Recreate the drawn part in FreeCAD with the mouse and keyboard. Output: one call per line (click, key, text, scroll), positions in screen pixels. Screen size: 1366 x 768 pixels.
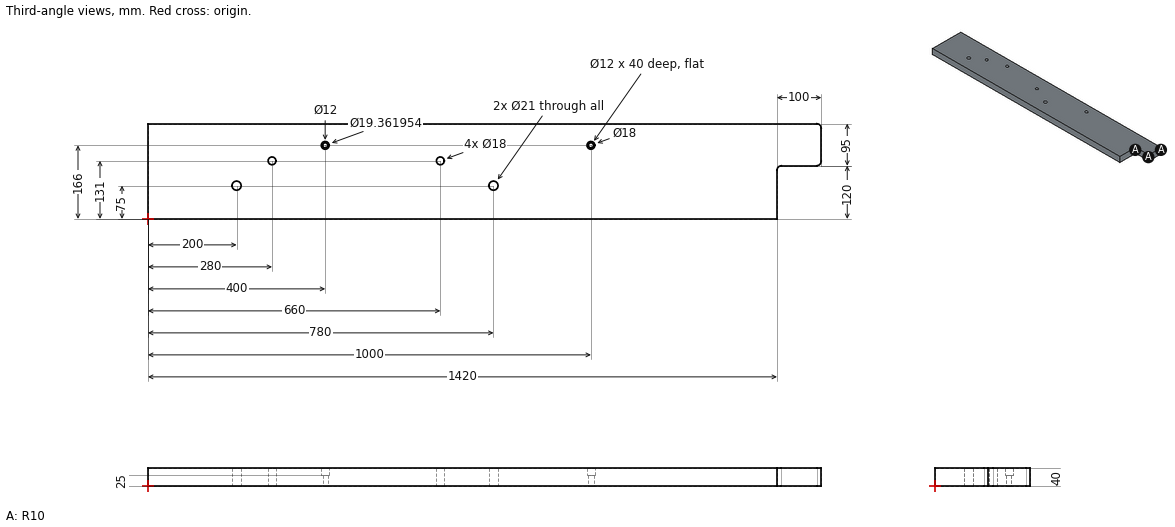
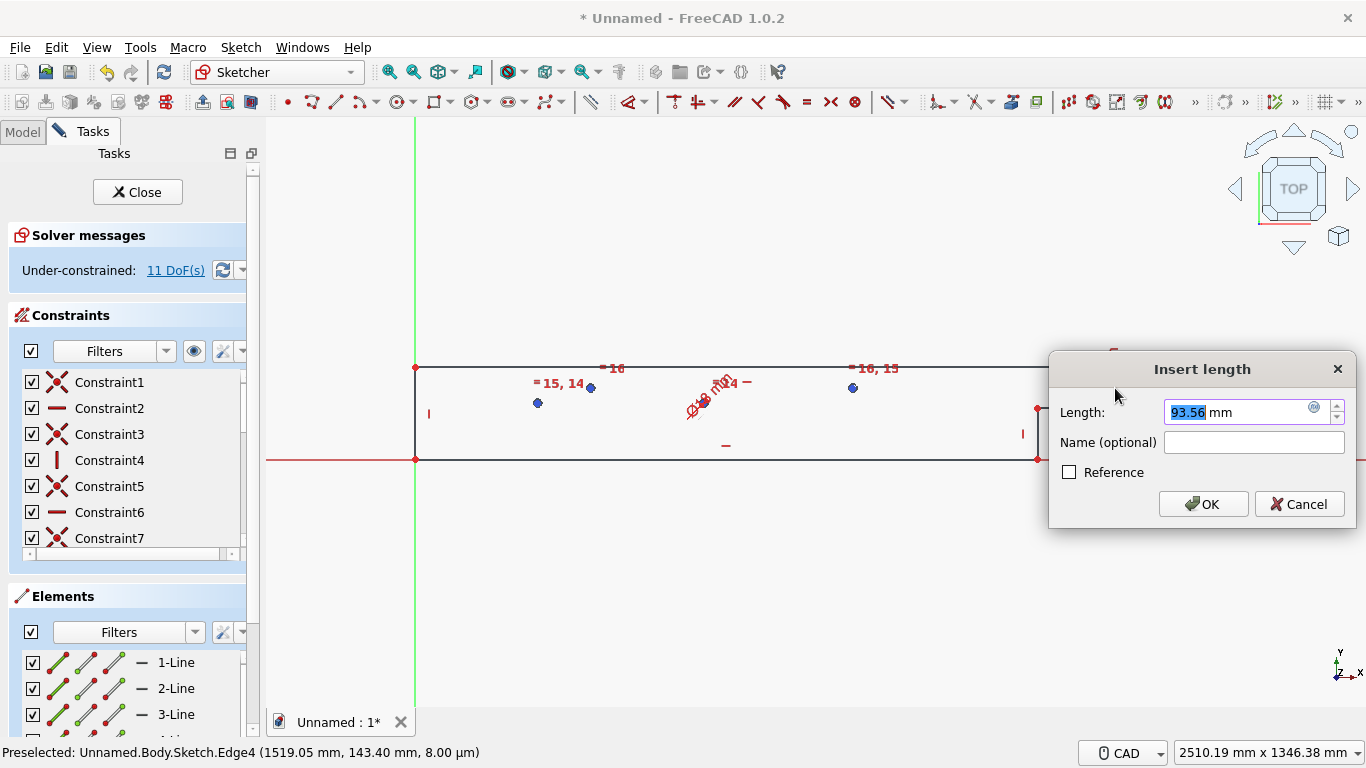
text(95)
key(Return)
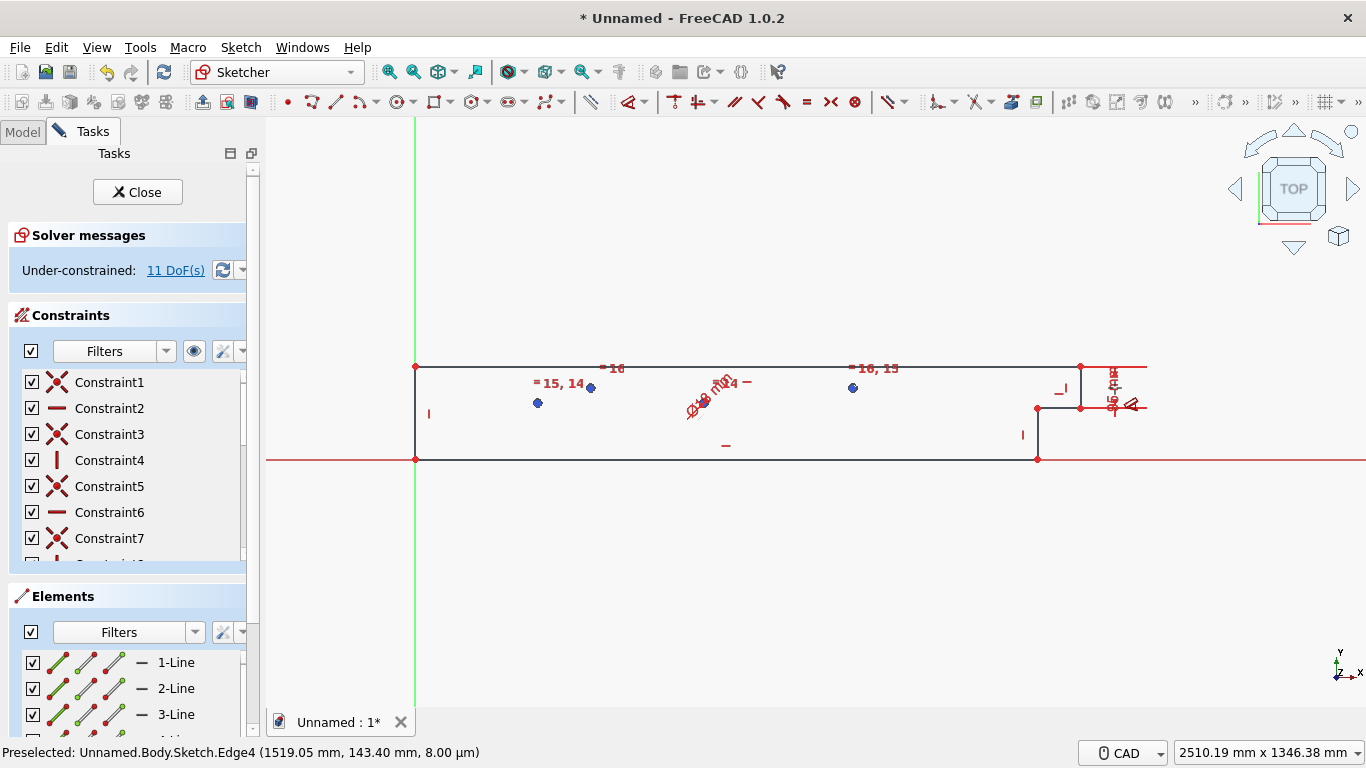
click(1038, 444)
click(1072, 434)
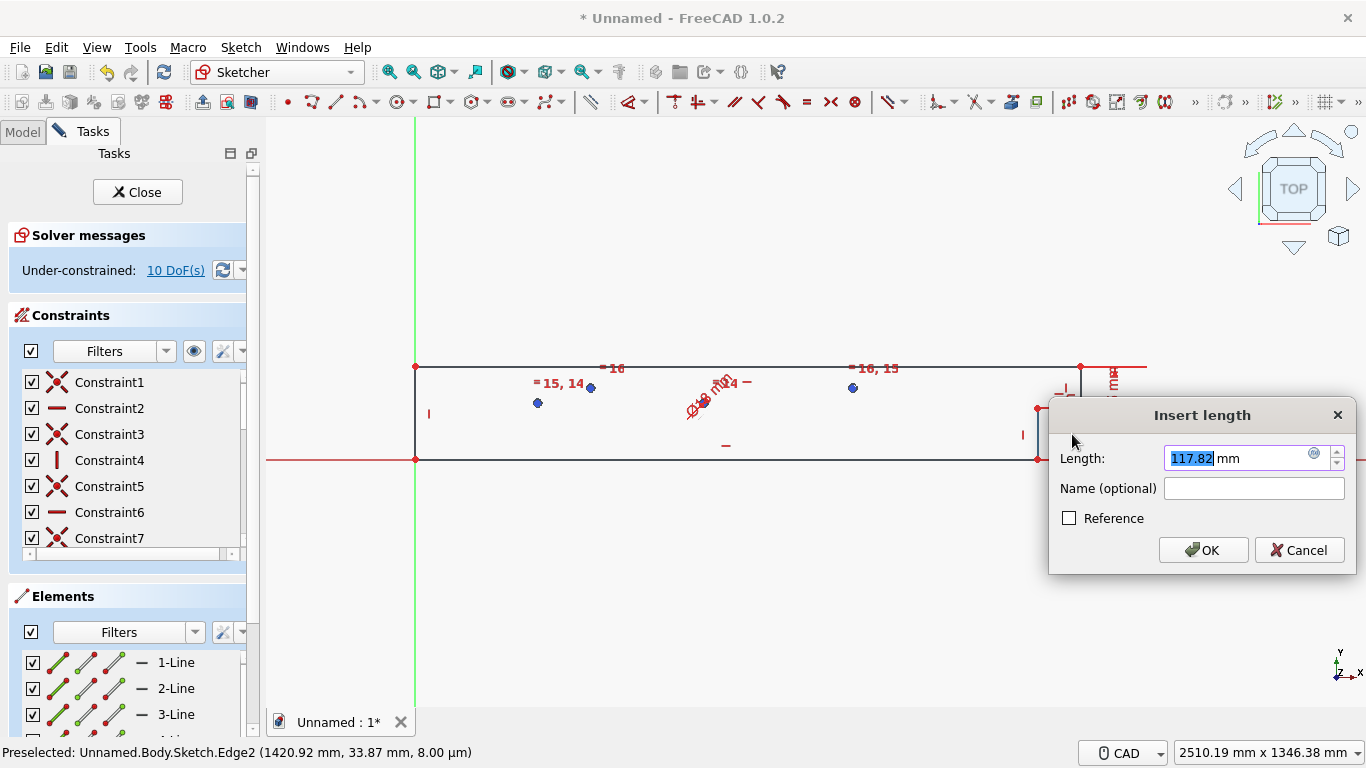
text(120)
key(Return)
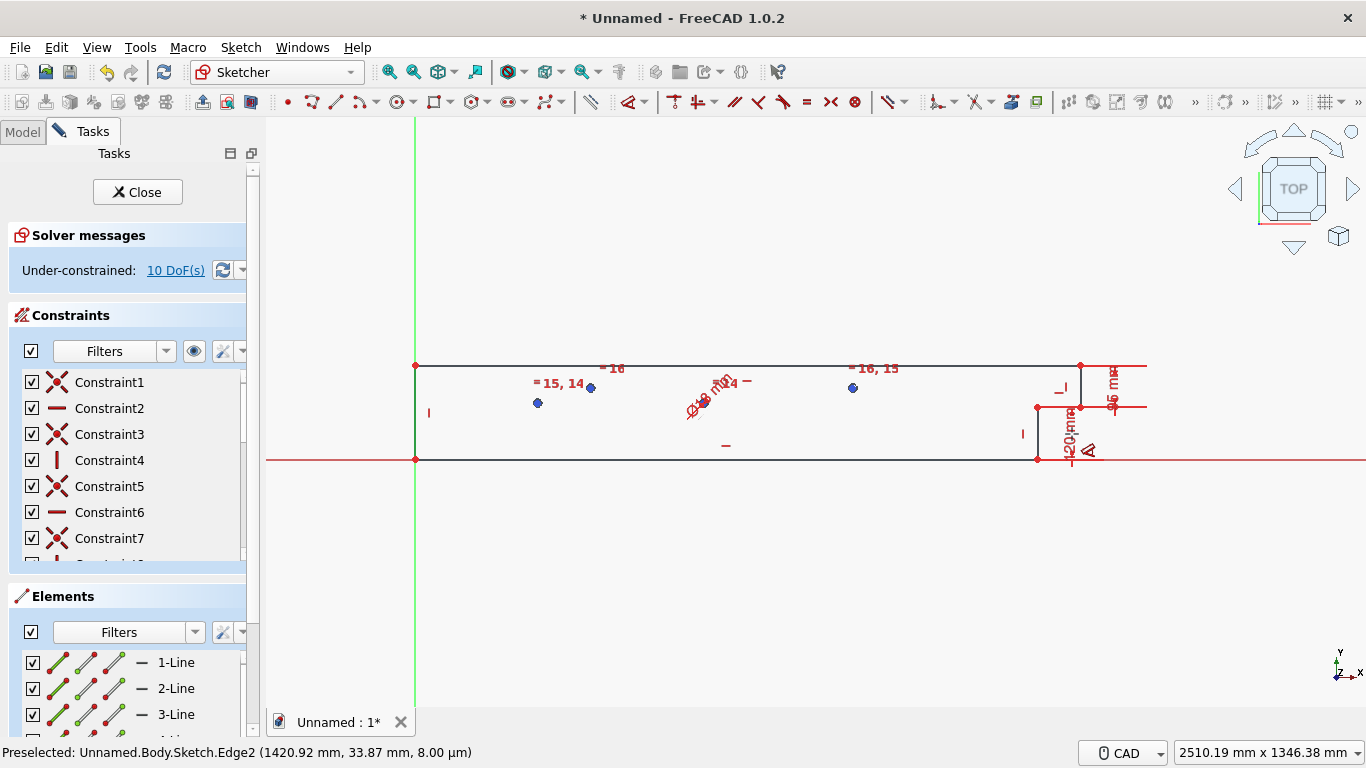
click(1051, 407)
click(1059, 349)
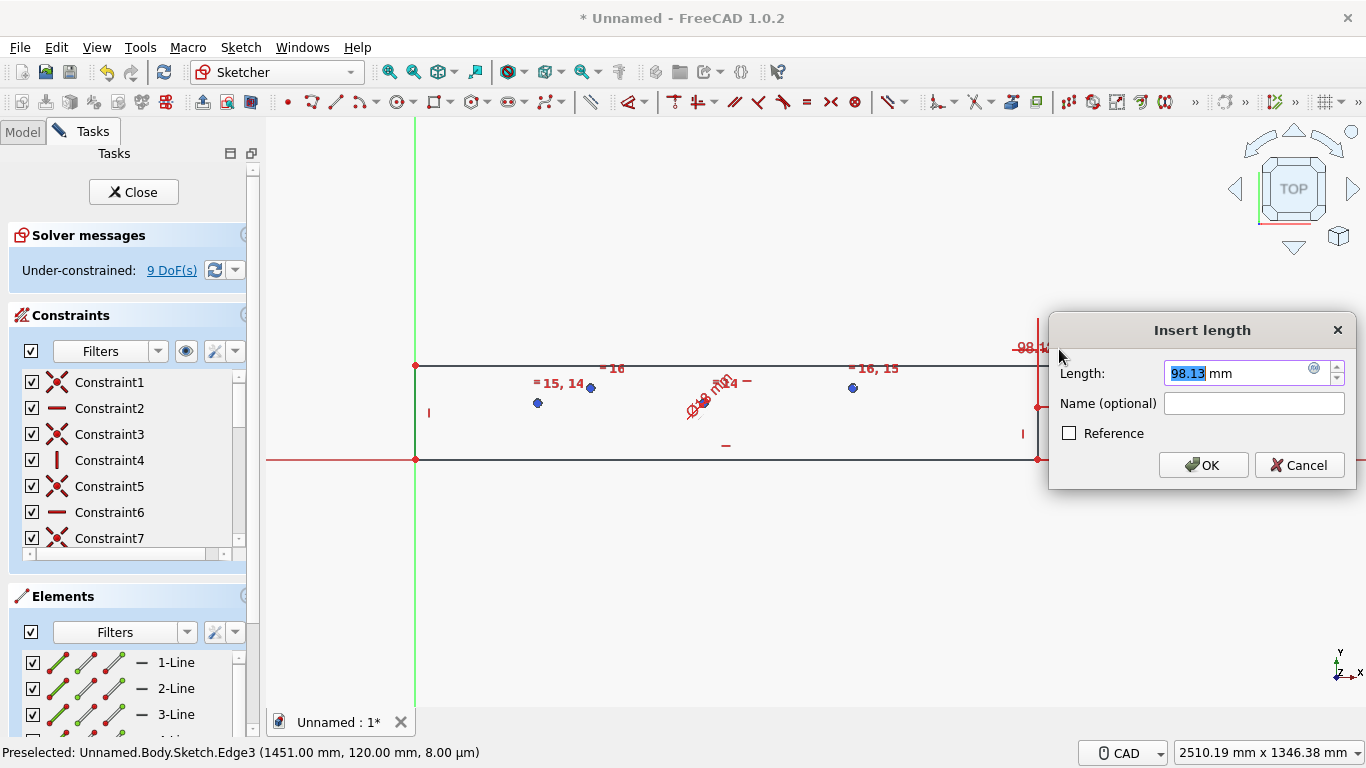
text(100)
key(Return)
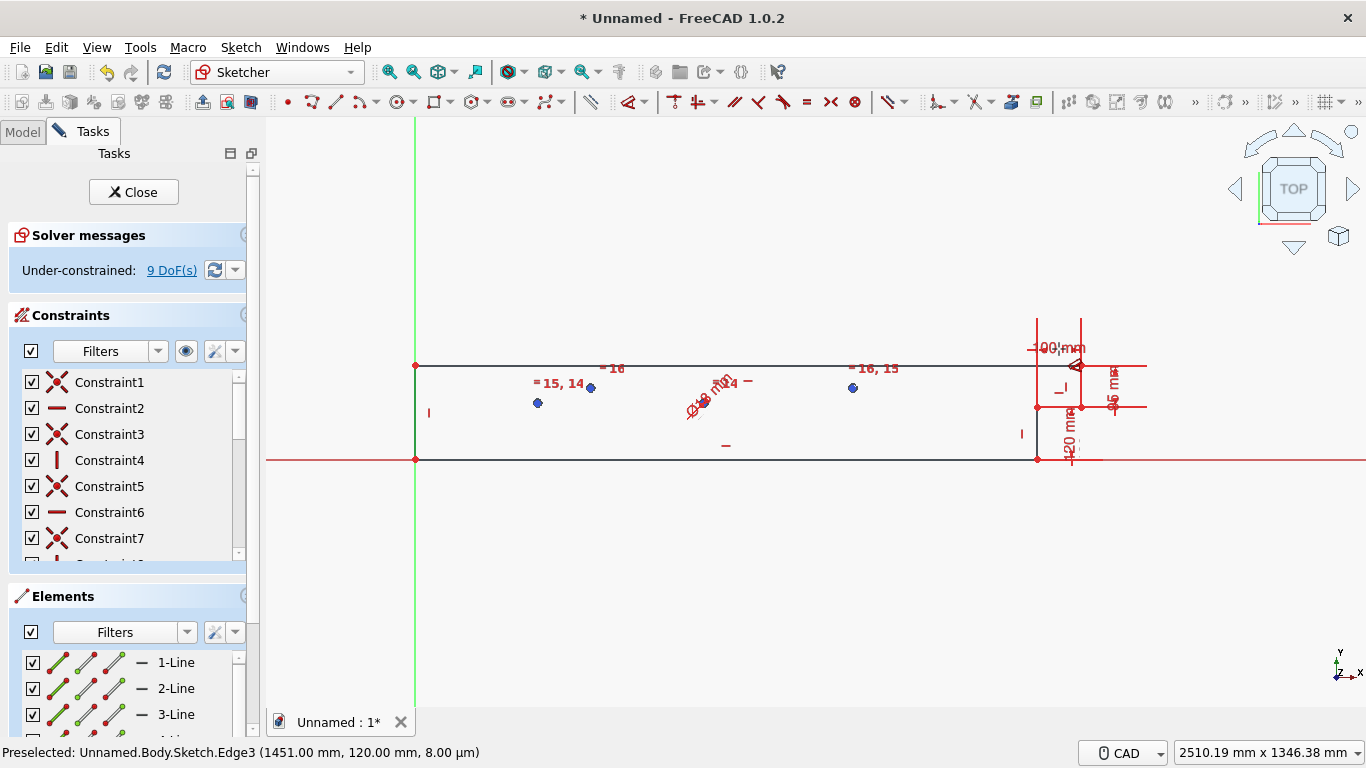
click(704, 403)
click(560, 494)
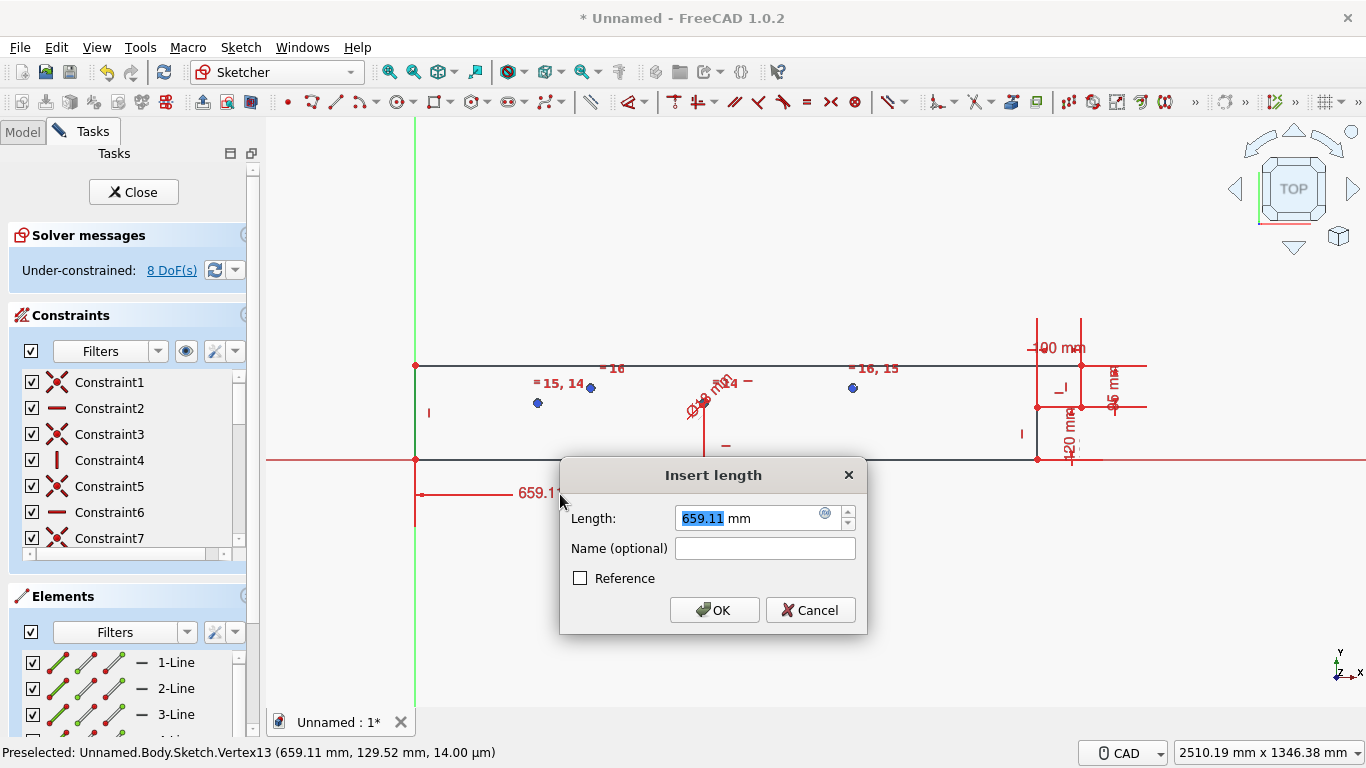
text(660)
key(Return)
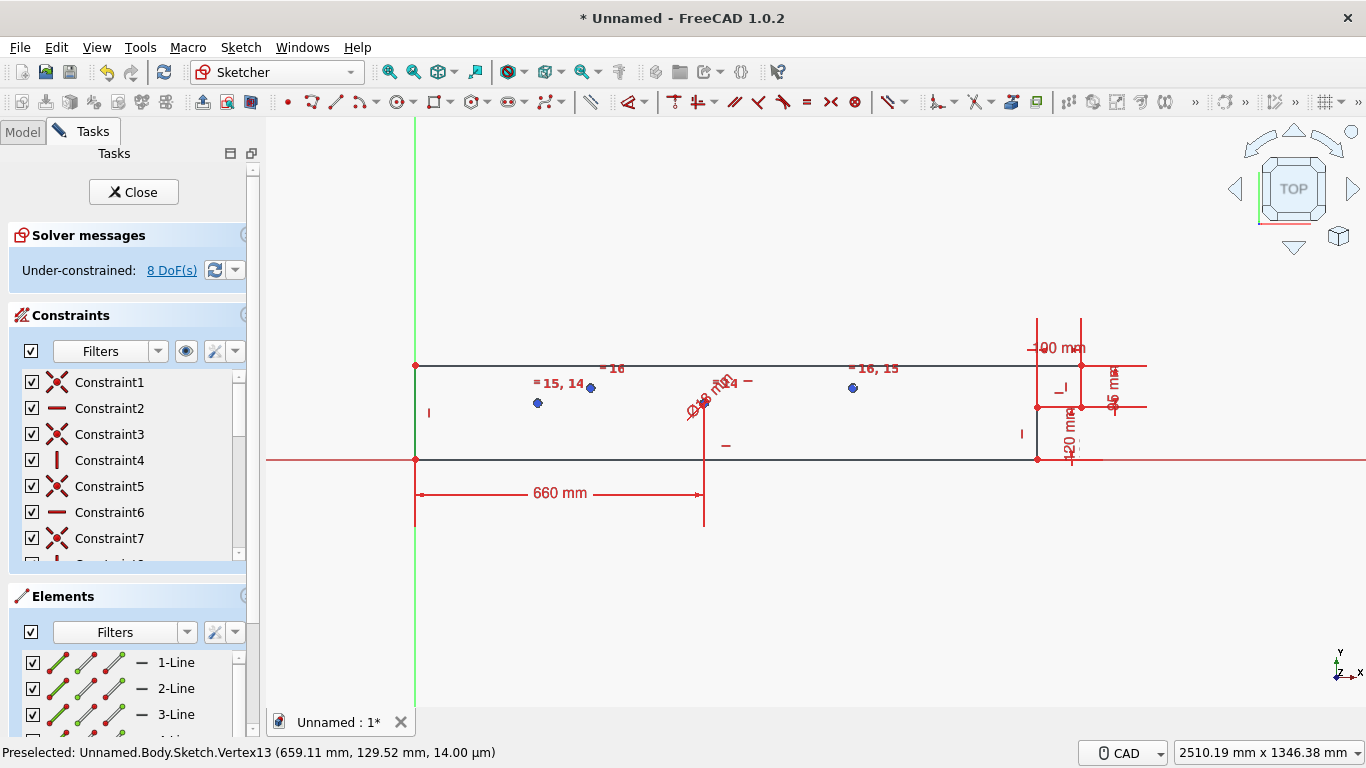
click(704, 403)
click(381, 431)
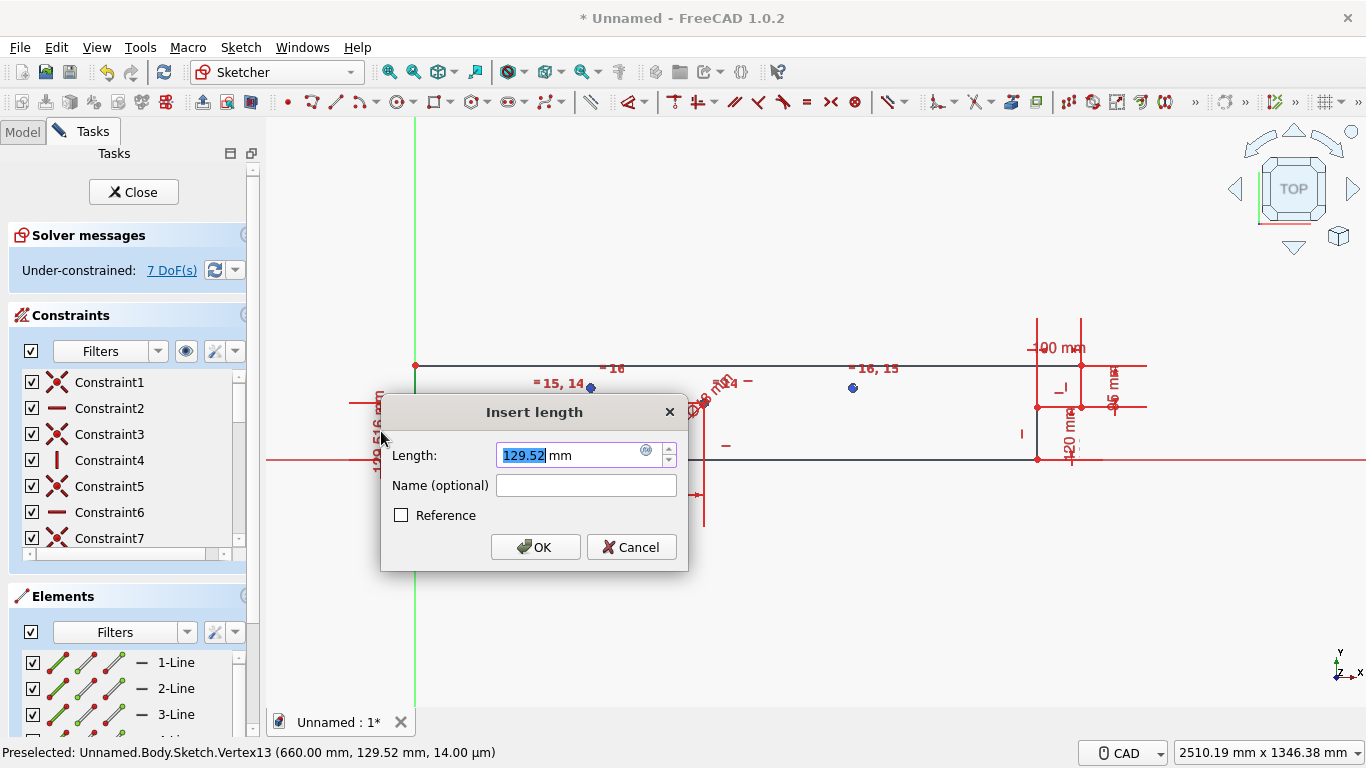
text(131)
key(Return)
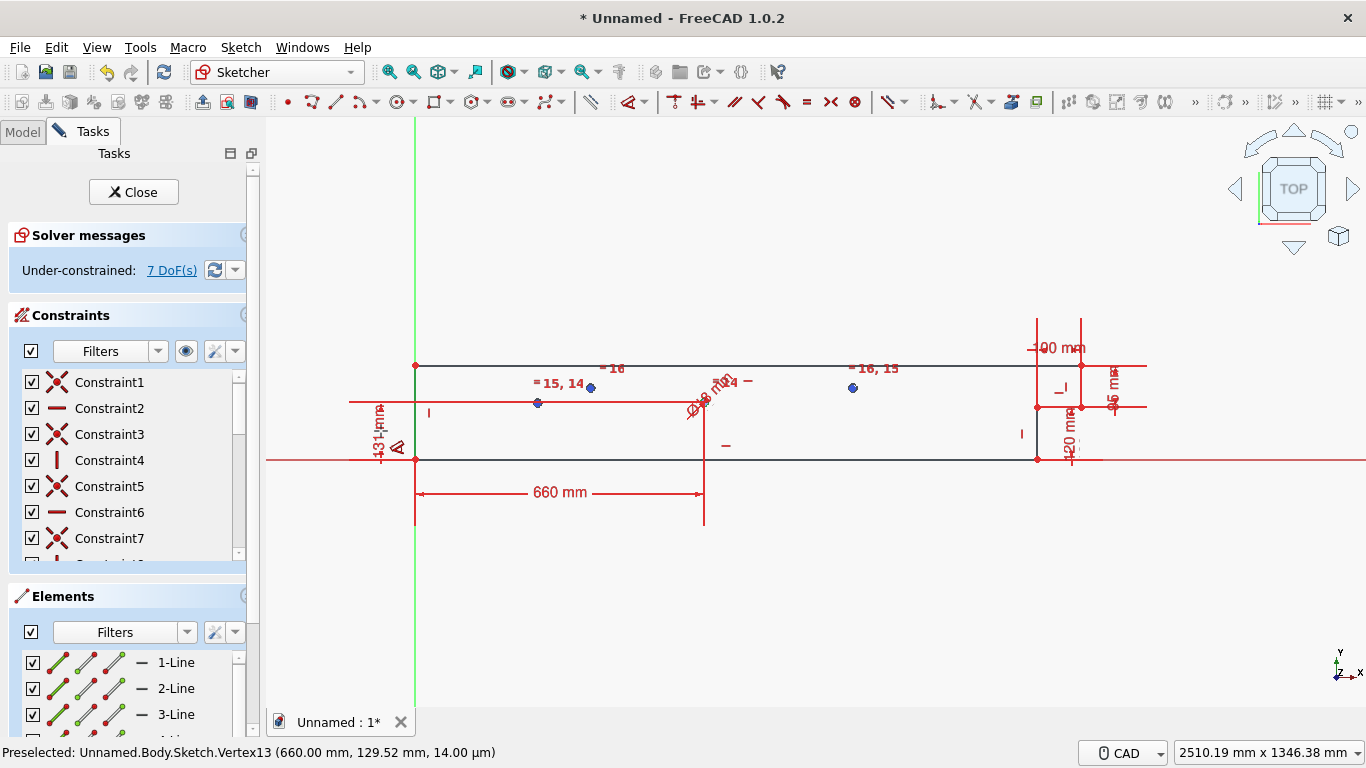
click(538, 403)
click(476, 494)